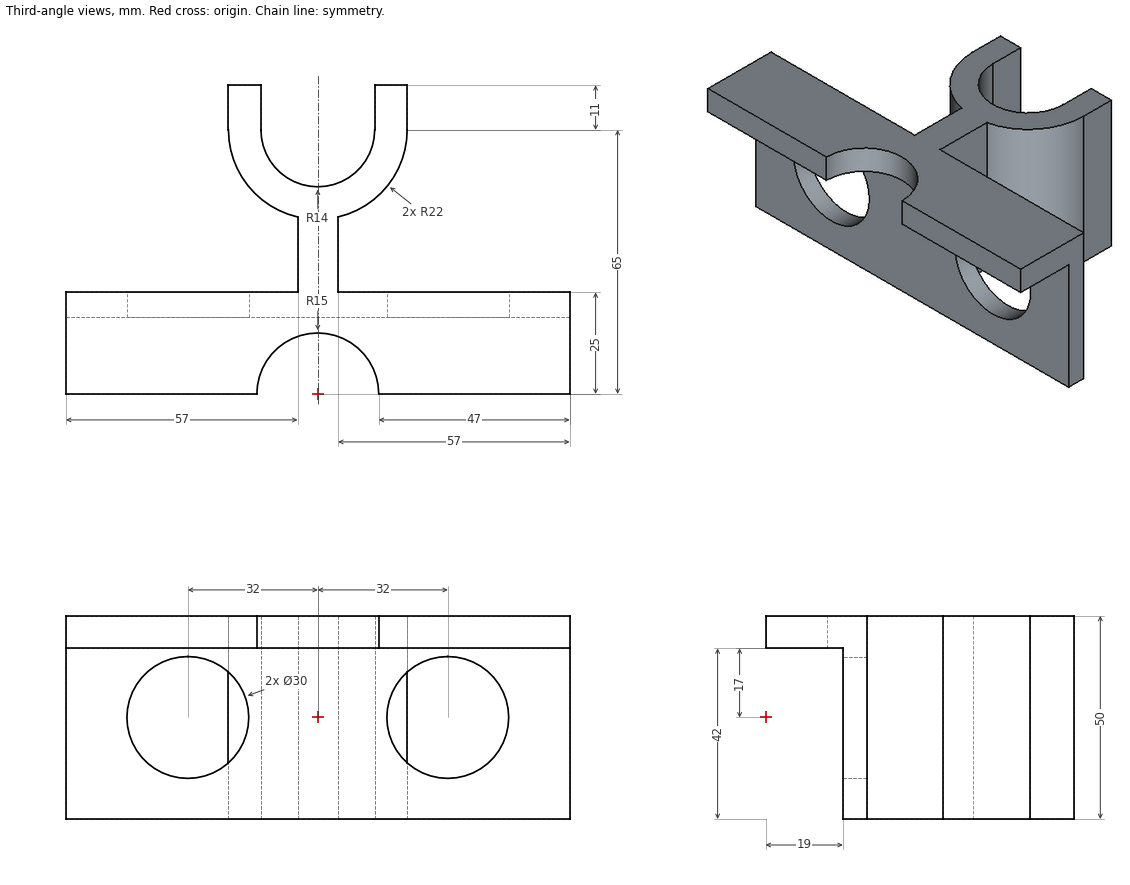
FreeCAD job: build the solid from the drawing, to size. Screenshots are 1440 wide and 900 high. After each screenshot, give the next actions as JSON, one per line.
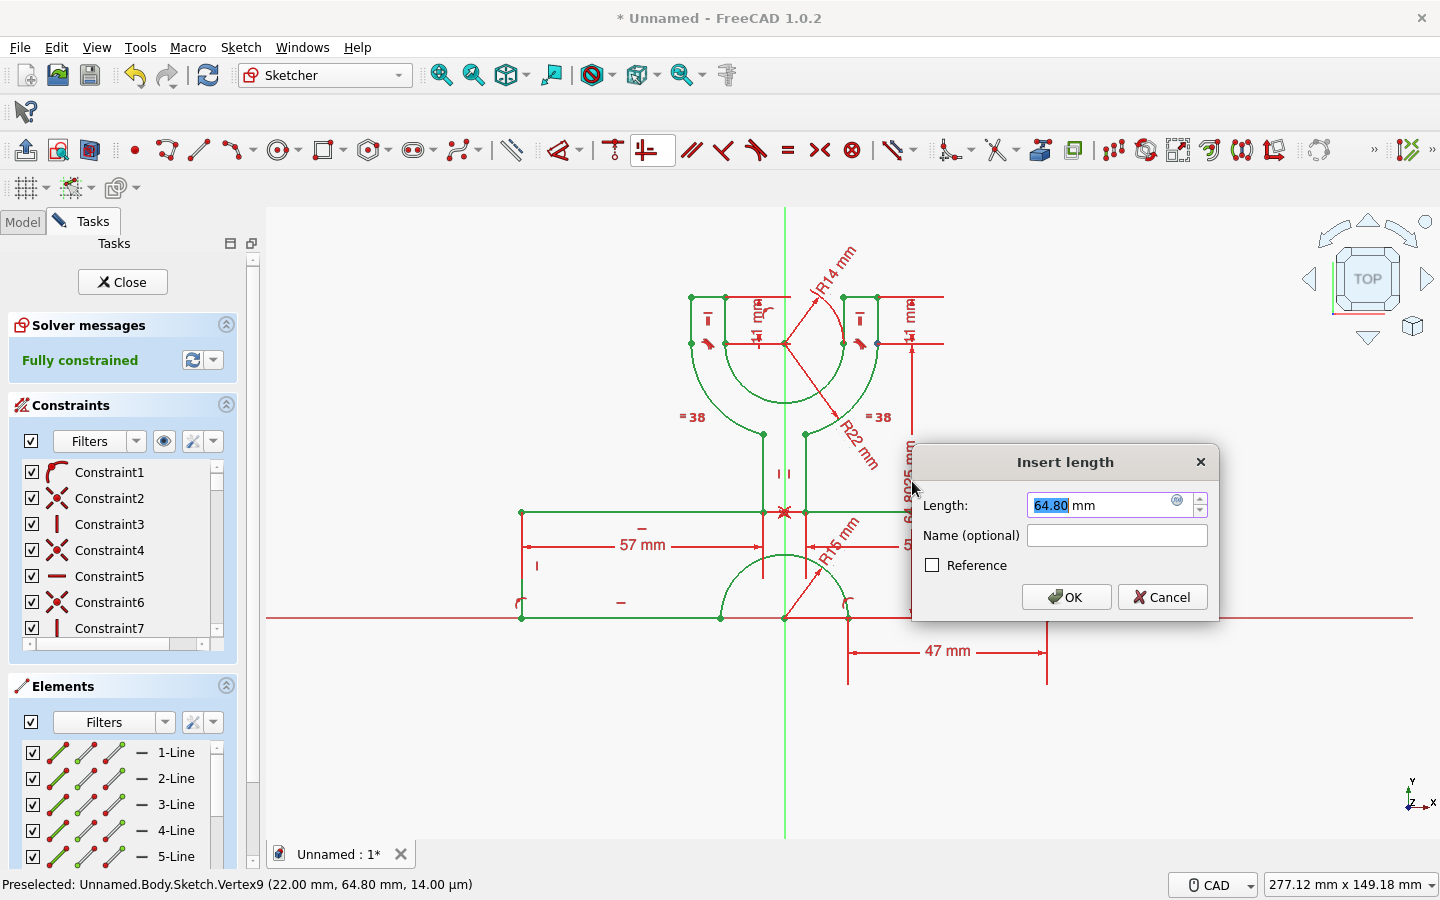
{"action": "type", "text": "65"}
{"action": "key", "text": "Return"}
{"action": "key", "text": "Escape"}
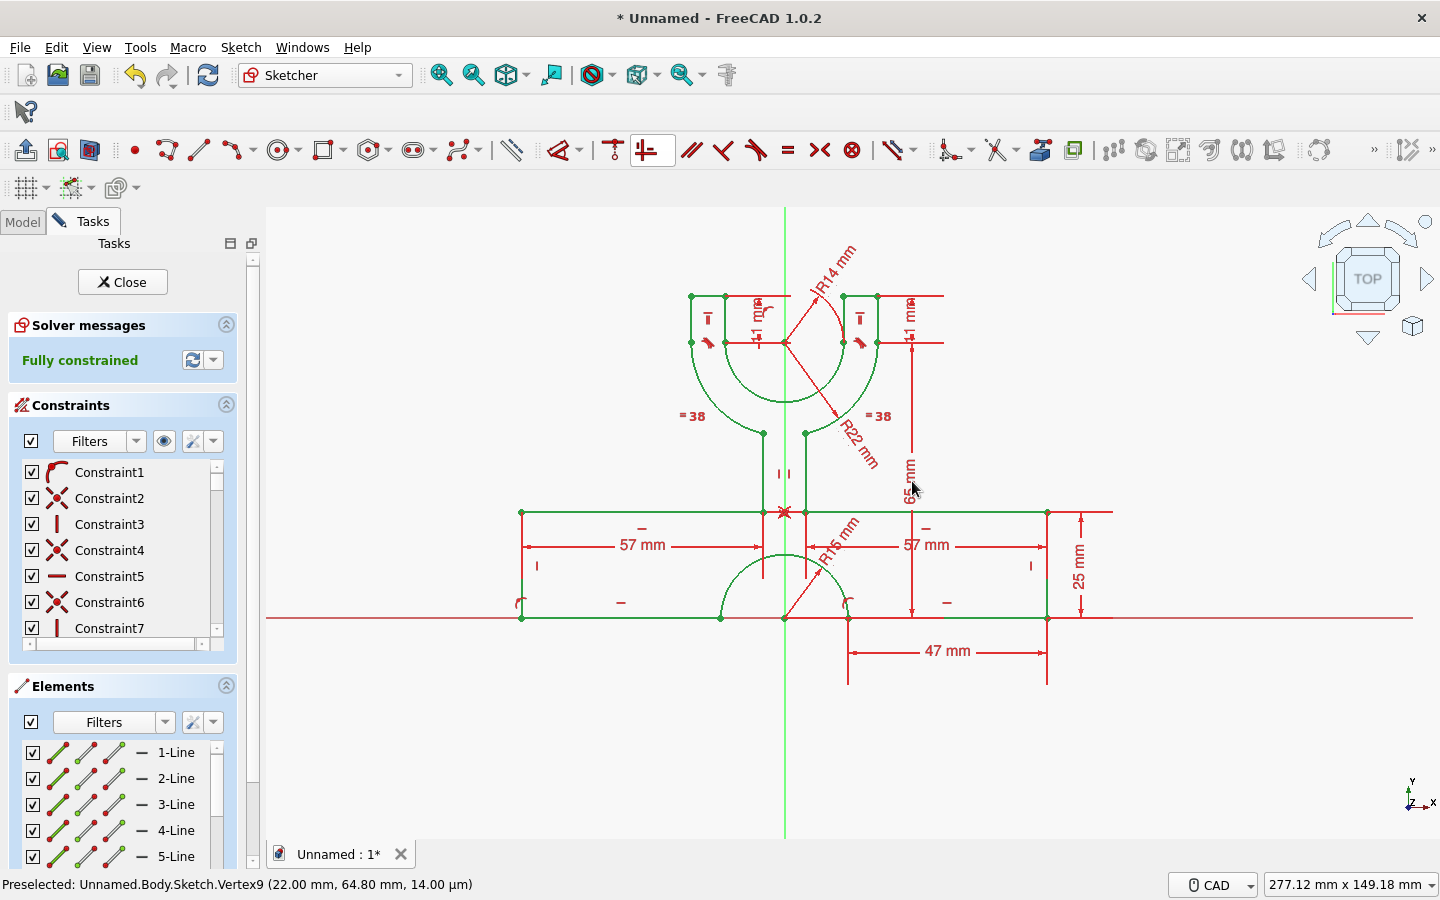
{"action": "left_click", "coordinate": [123, 282]}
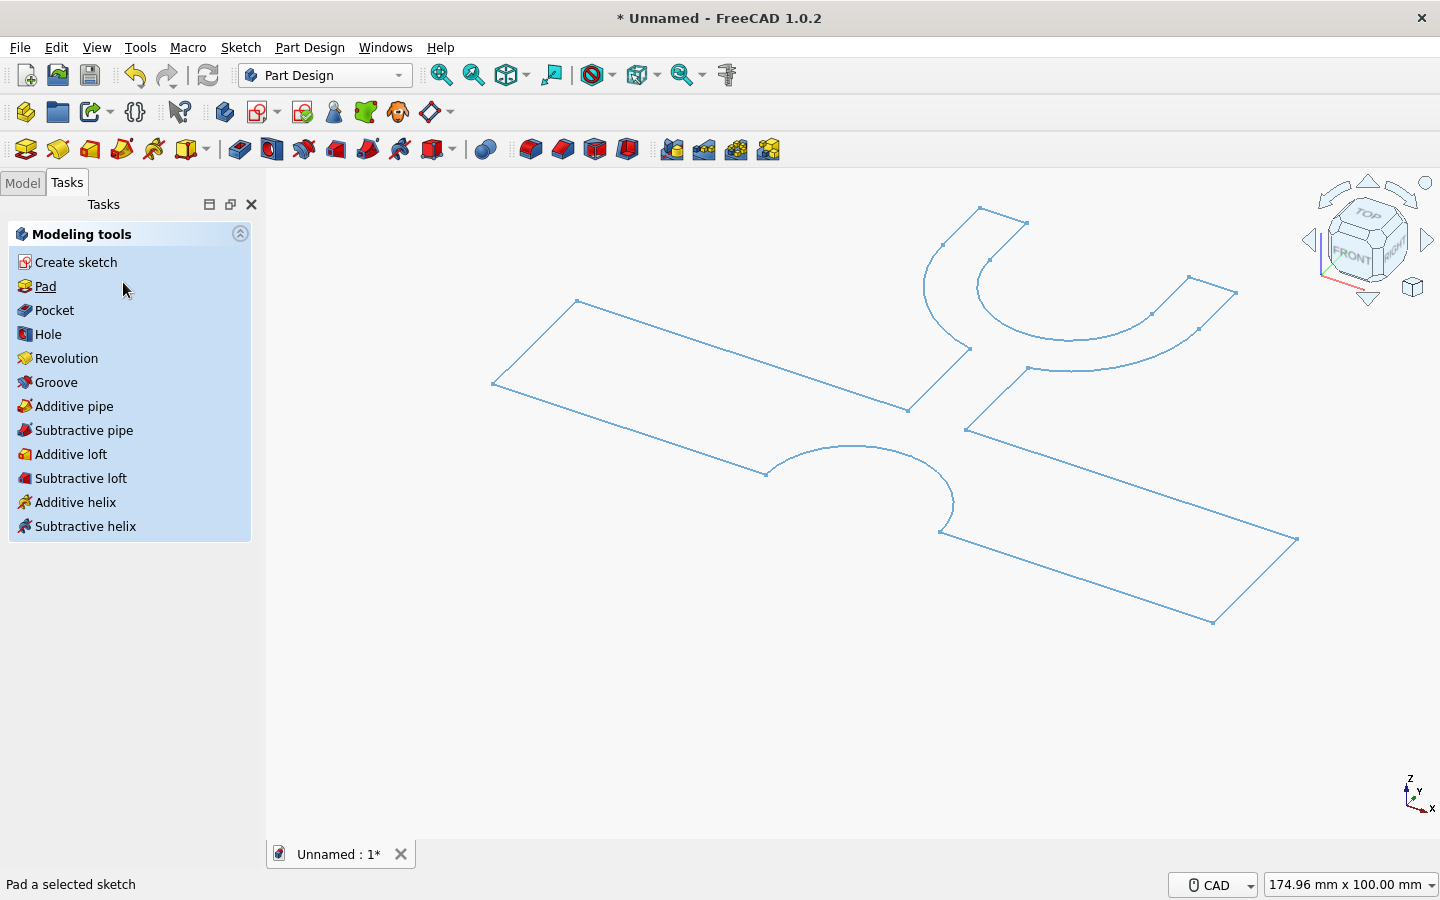
{"action": "left_click", "coordinate": [26, 150]}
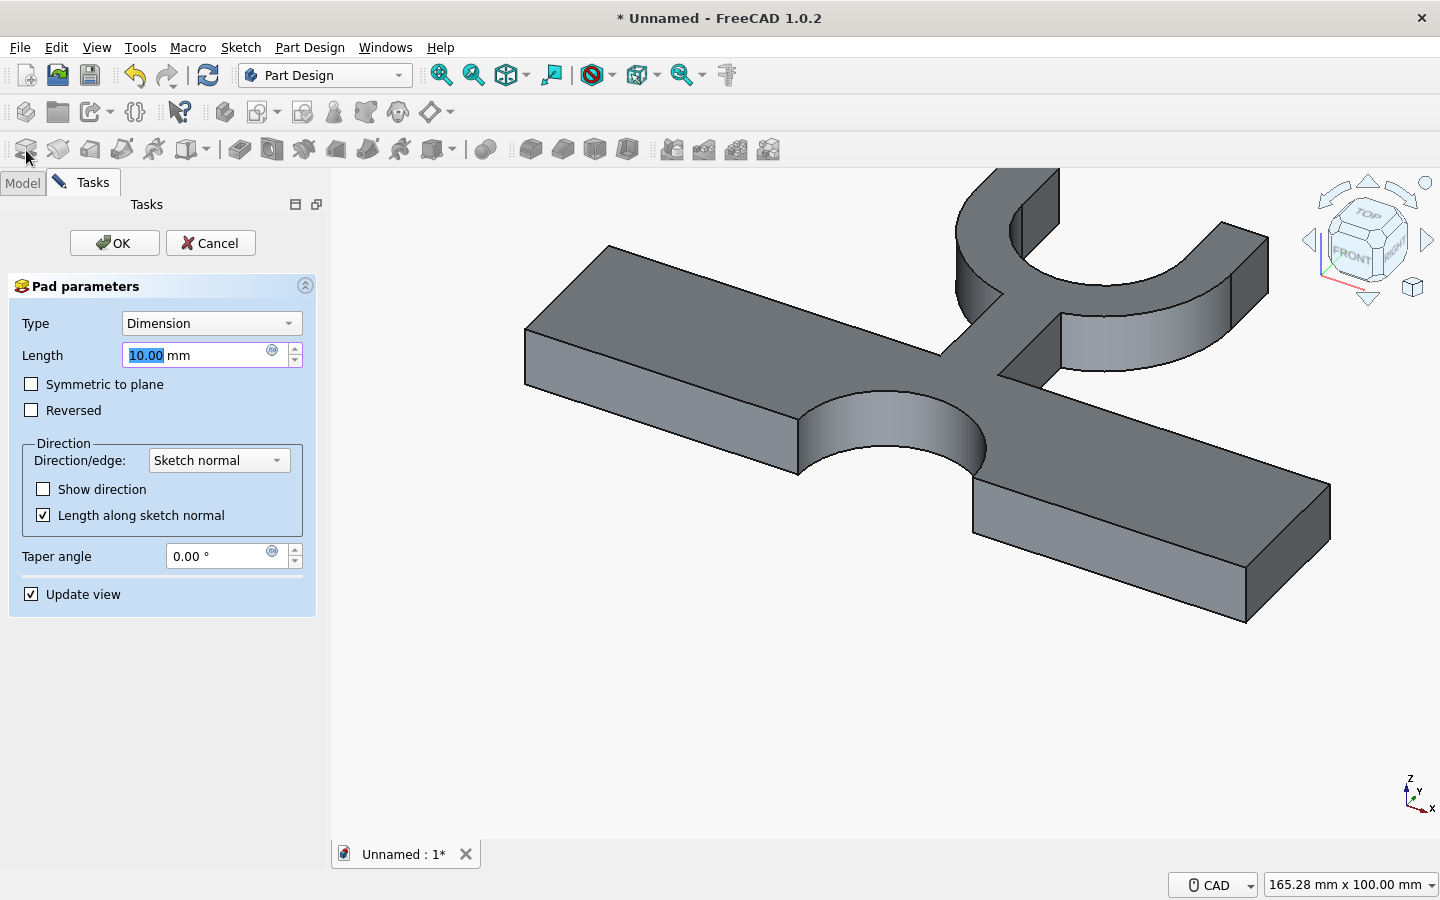
{"action": "type", "text": "50"}
{"action": "key", "text": "Tab"}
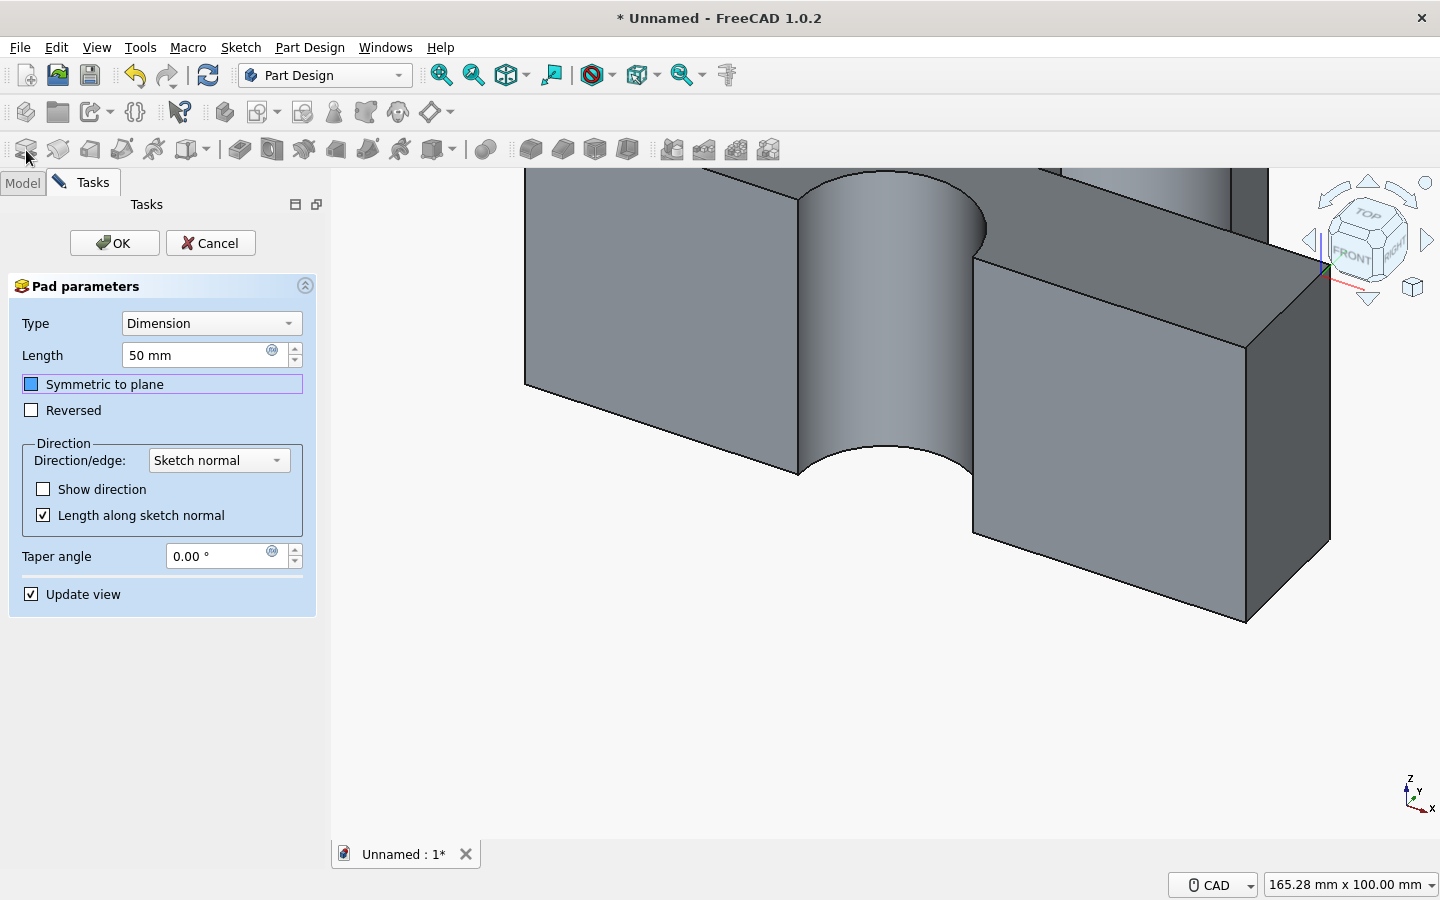
{"action": "left_click", "coordinate": [30, 384]}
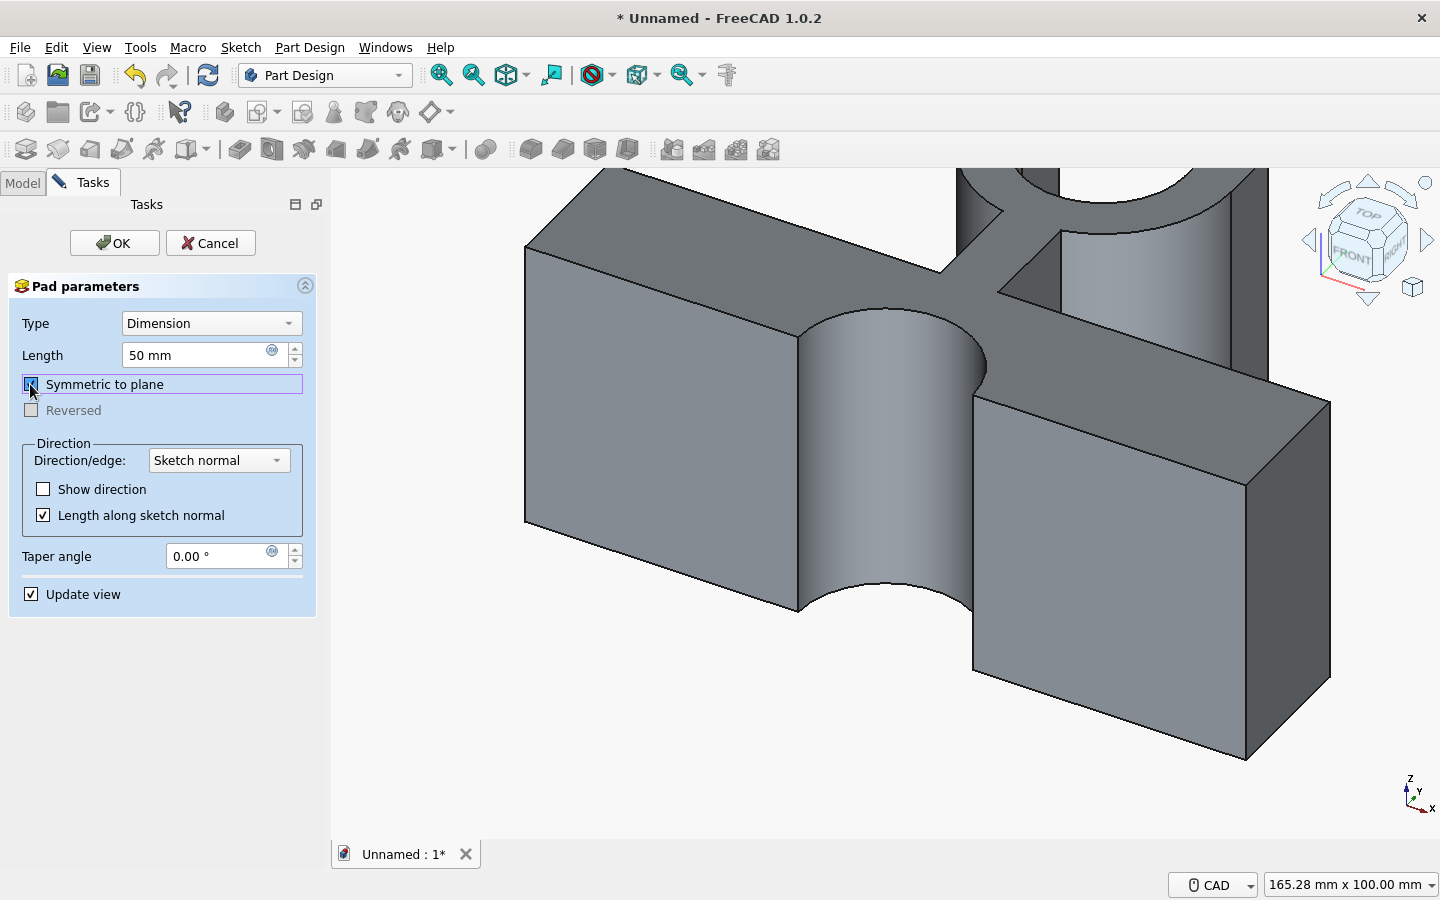
{"action": "left_click", "coordinate": [115, 243]}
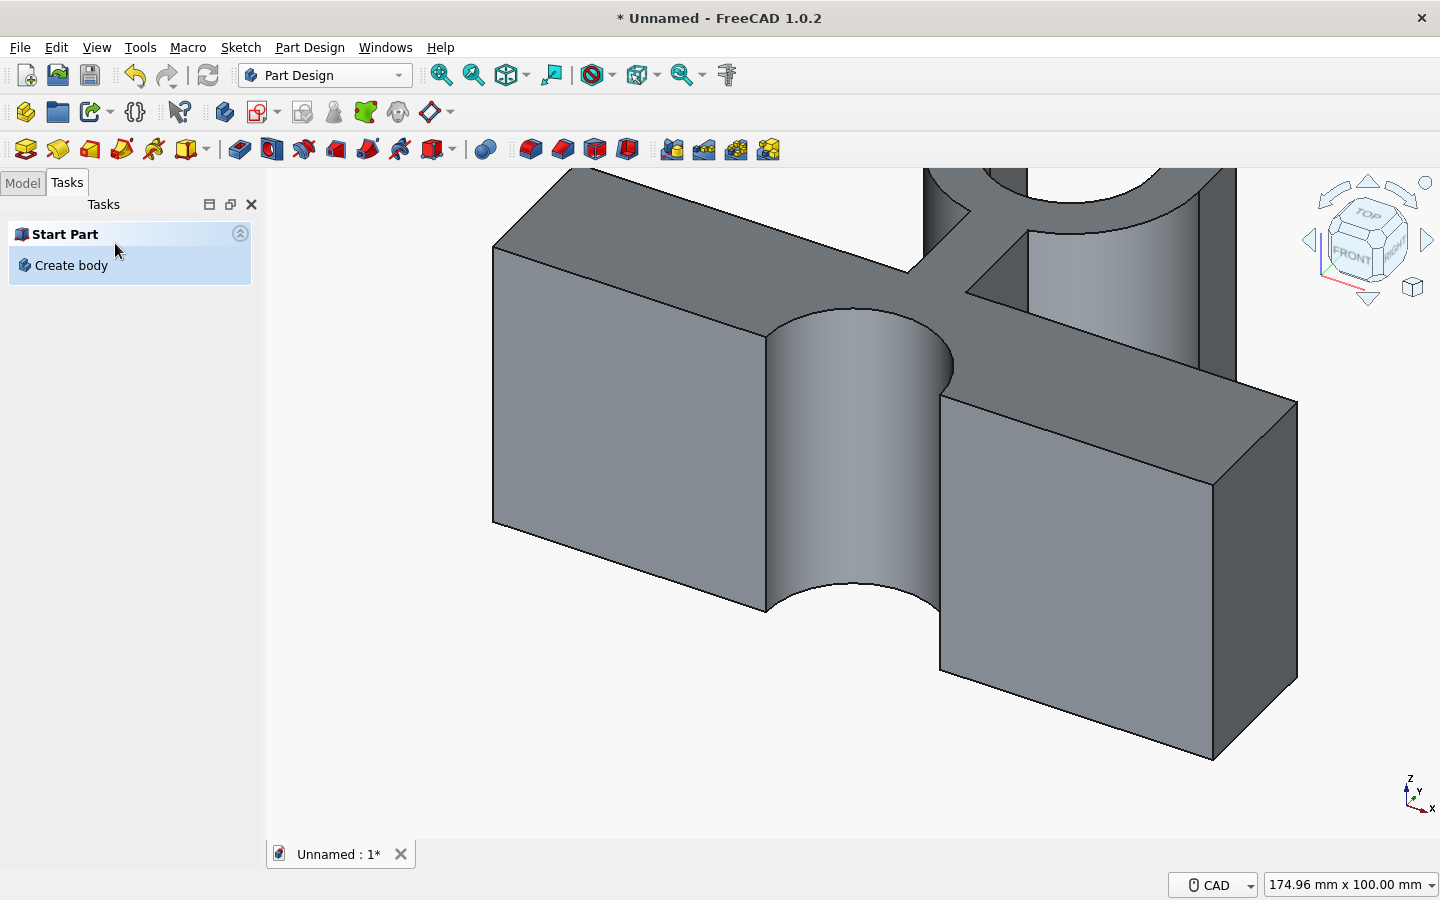
{"action": "left_click", "coordinate": [442, 76]}